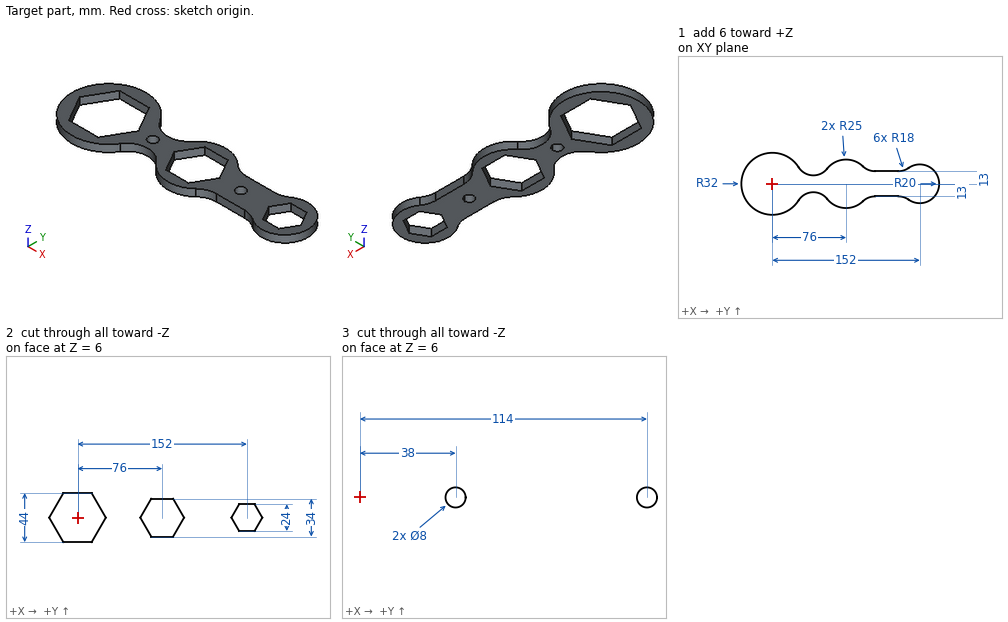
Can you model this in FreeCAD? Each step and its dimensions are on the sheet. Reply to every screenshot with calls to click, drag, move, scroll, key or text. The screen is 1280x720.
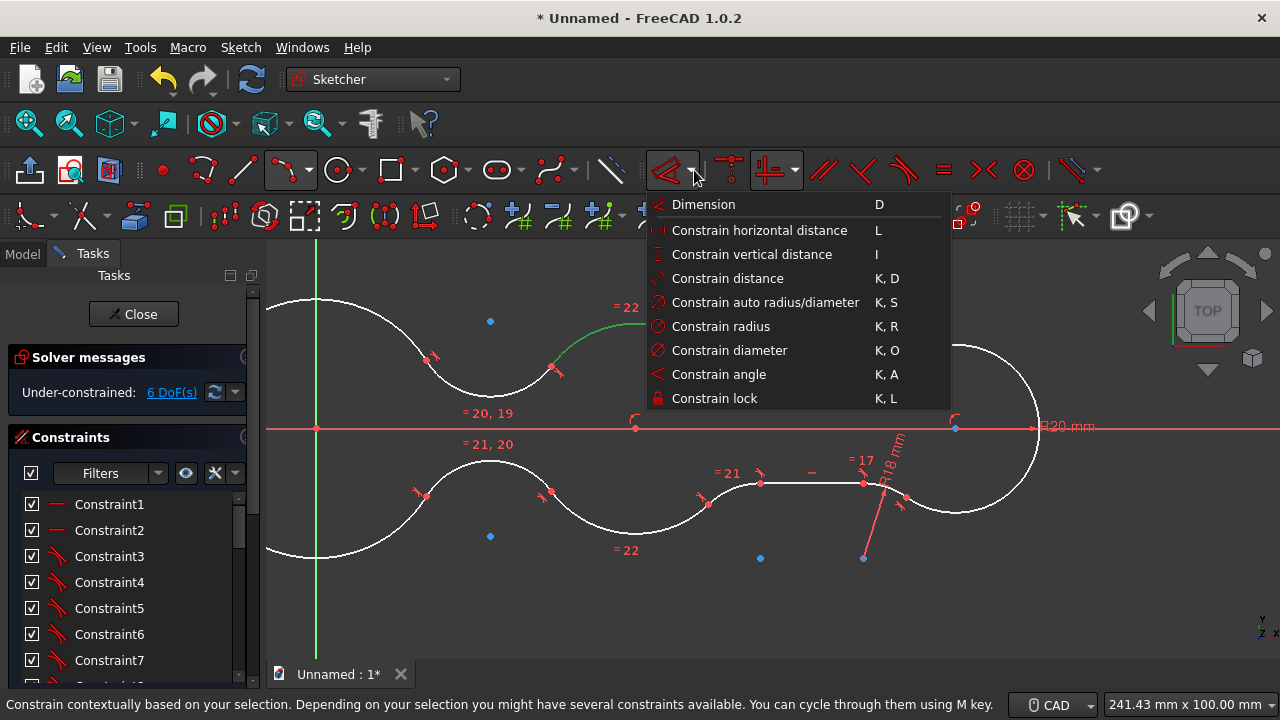
click(799, 326)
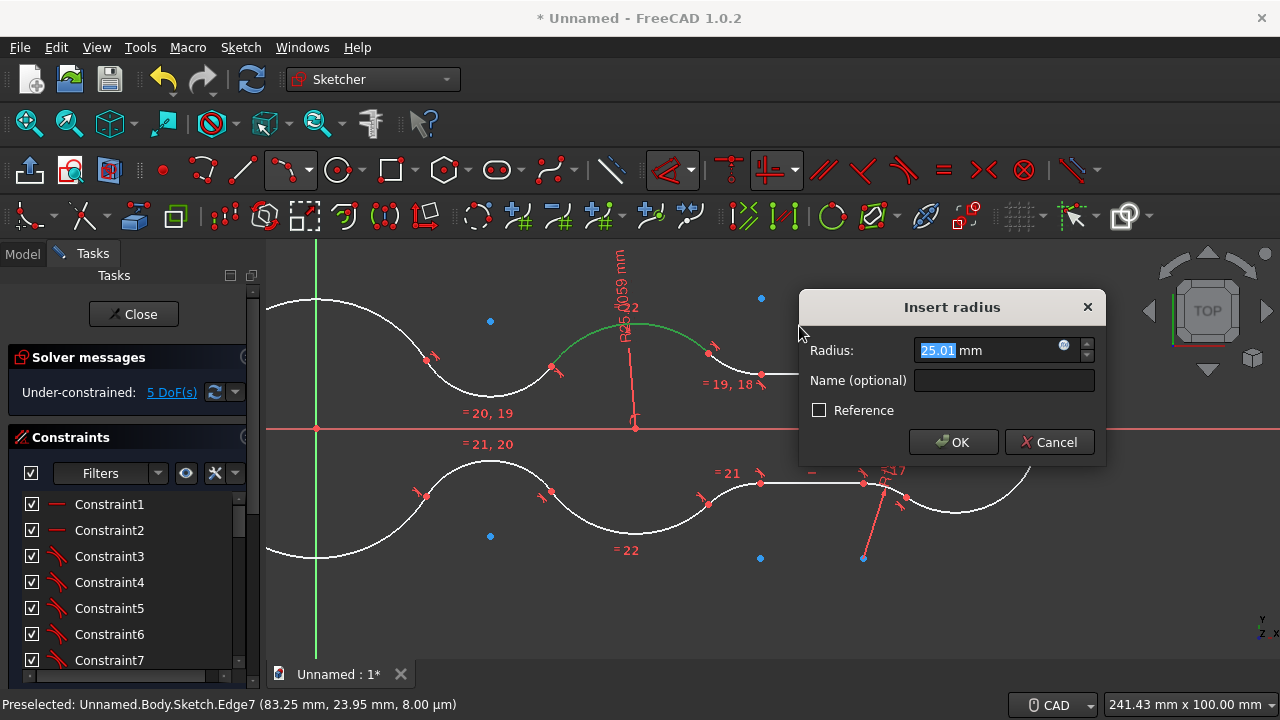
text(25)
key(Return)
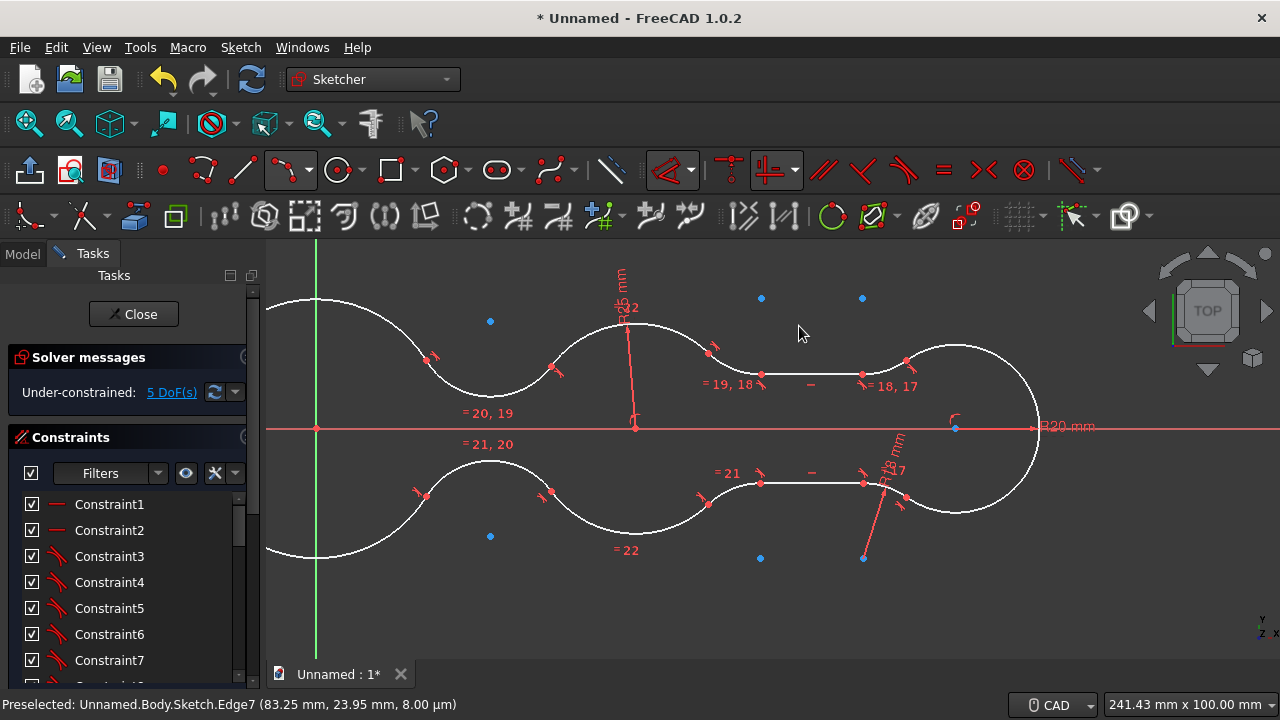
click(314, 299)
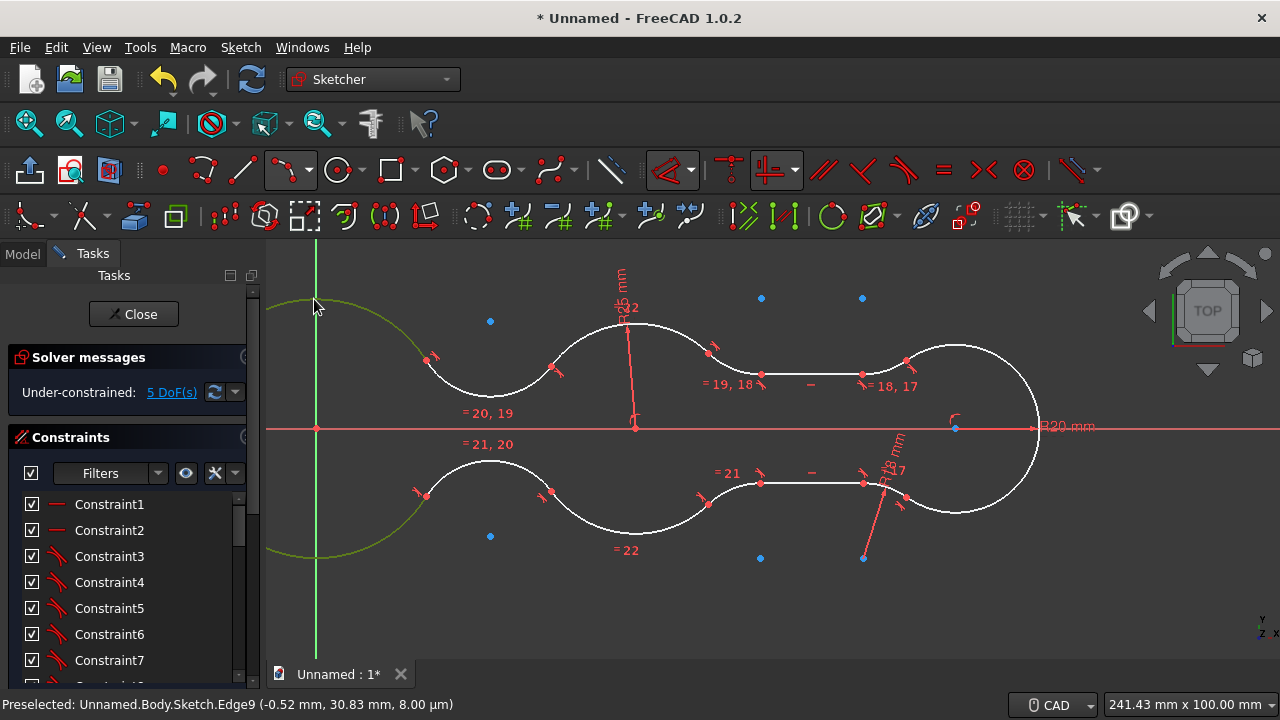
key(k)
key(r)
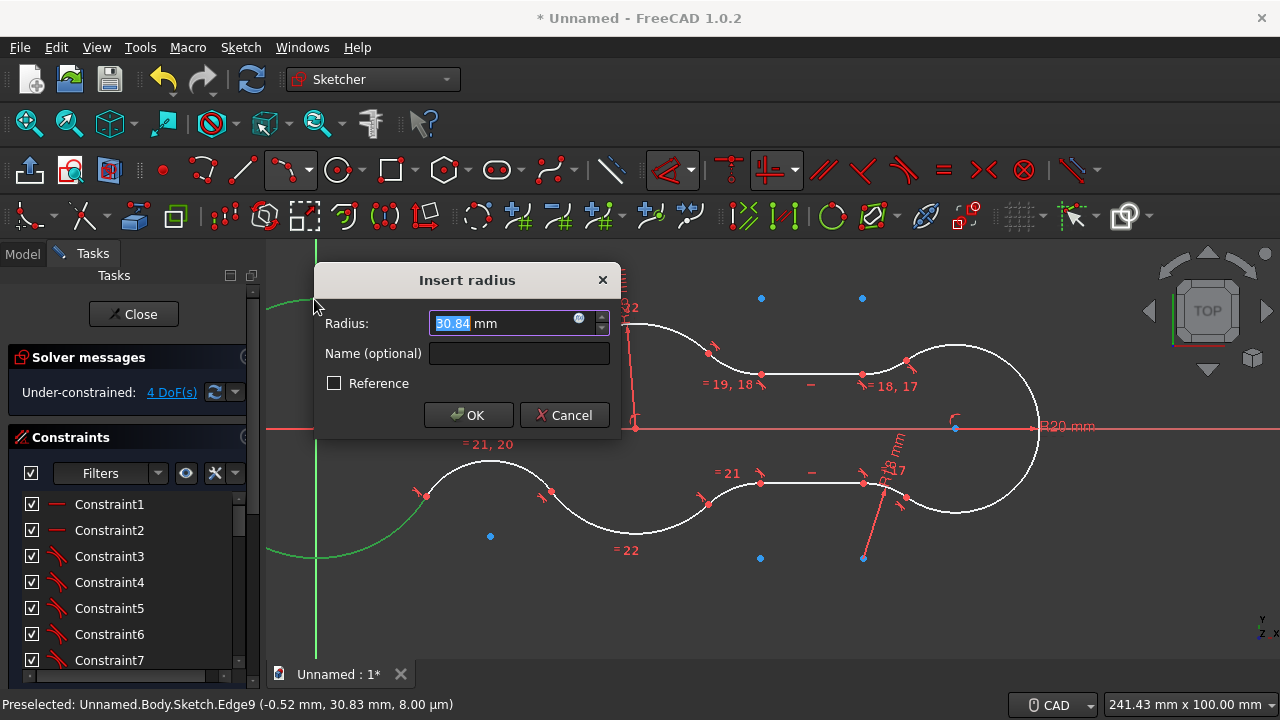
text(32)
key(Return)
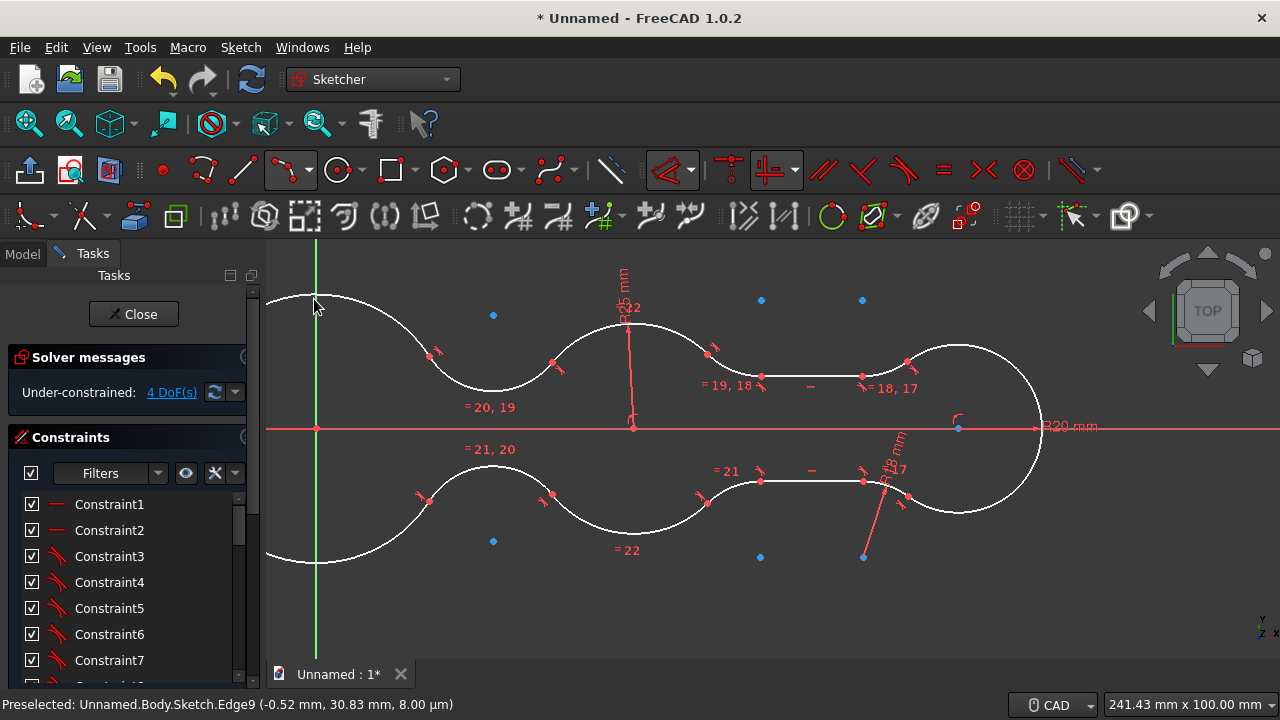
click(761, 481)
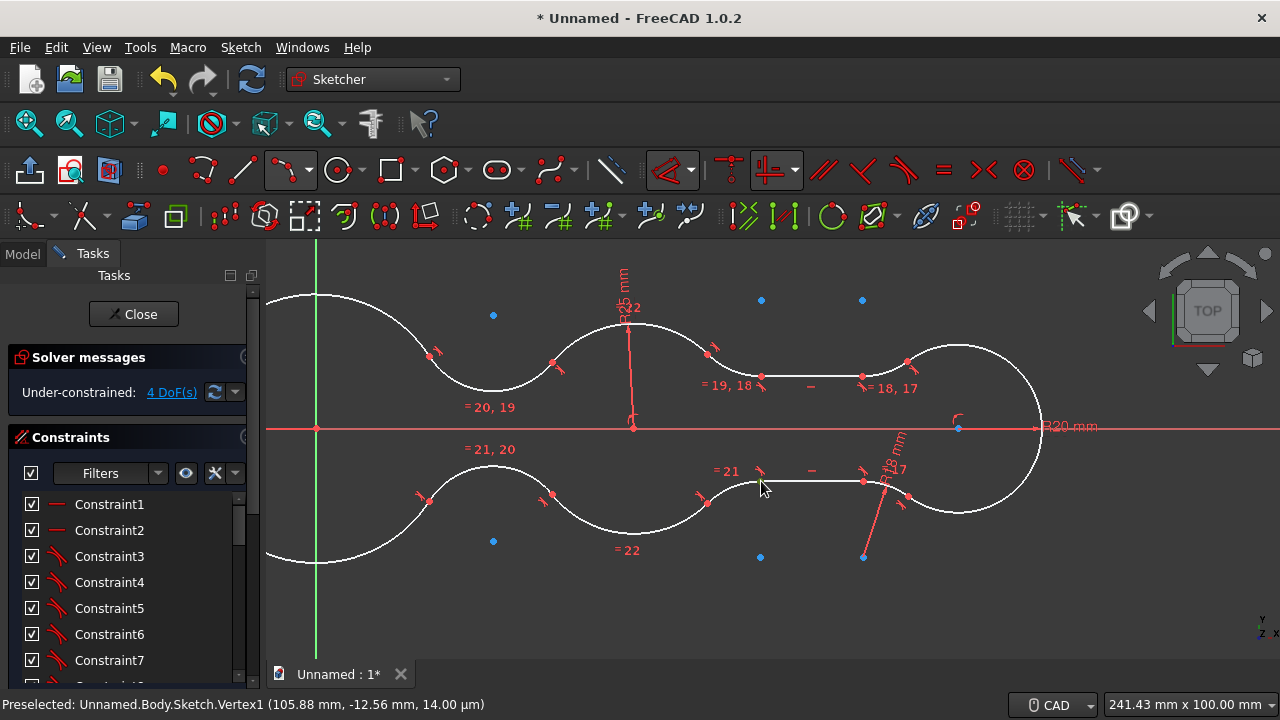
click(694, 170)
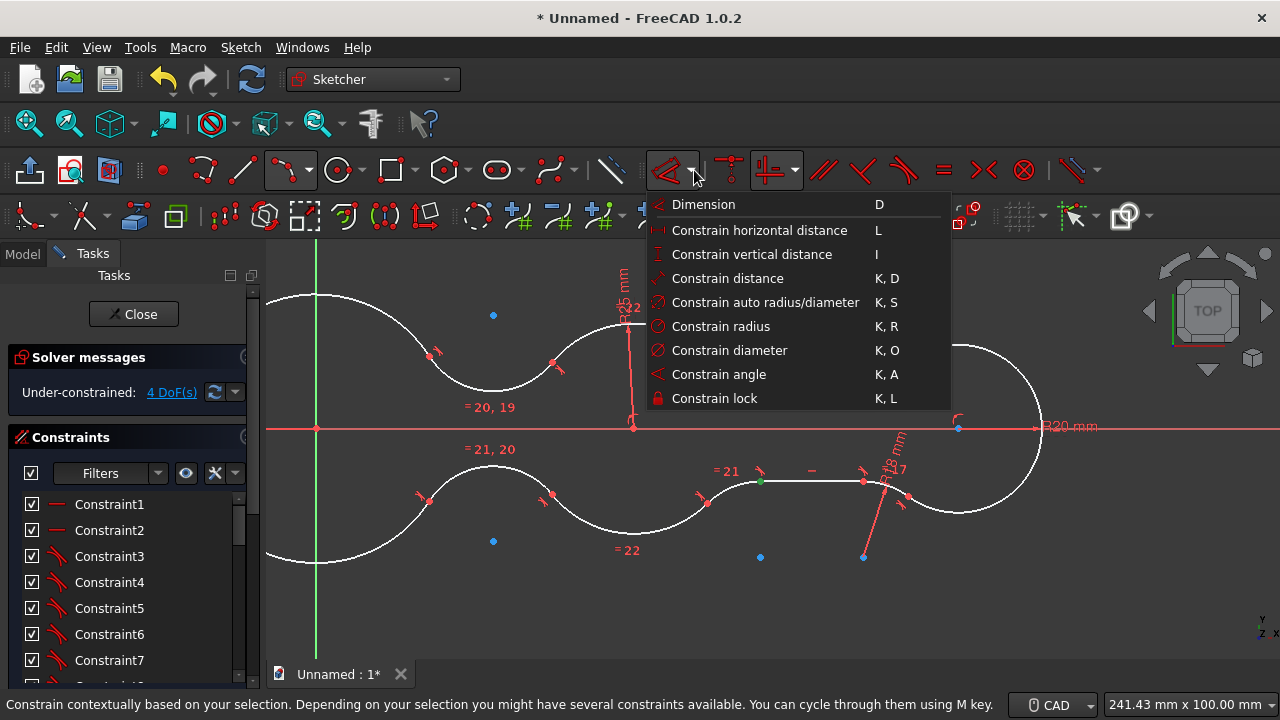
click(799, 254)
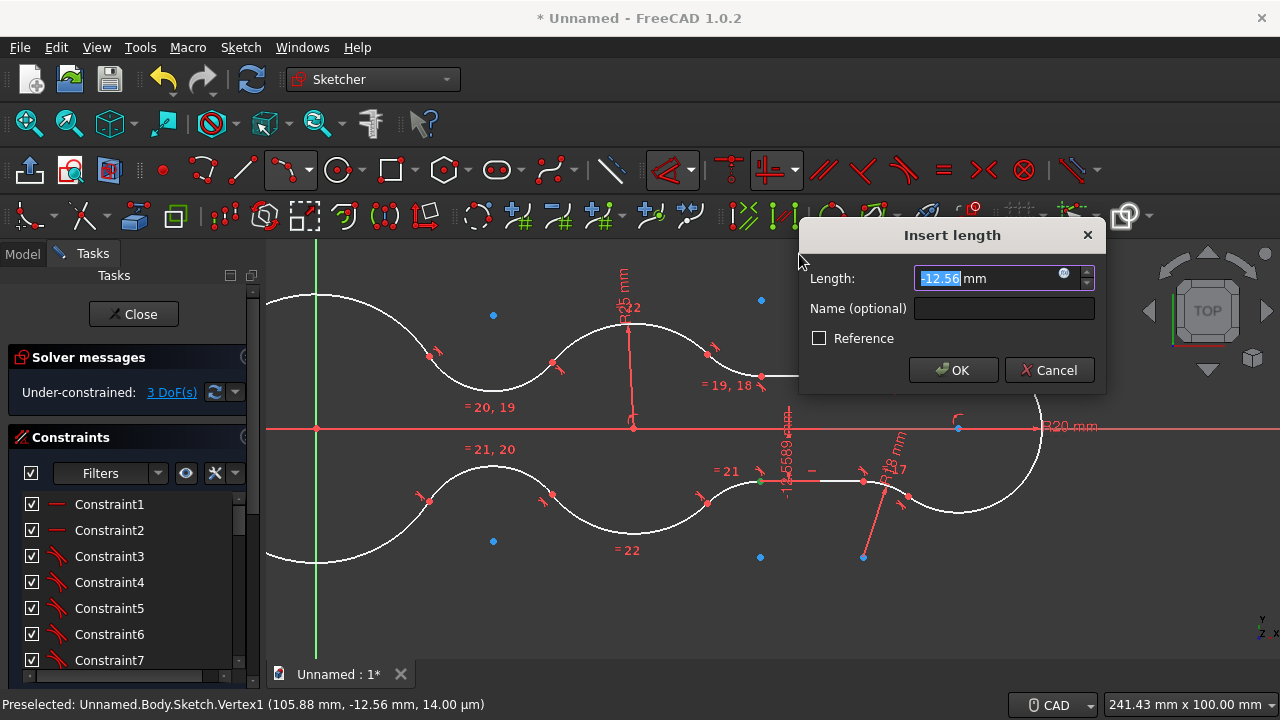
text(-13)
key(Return)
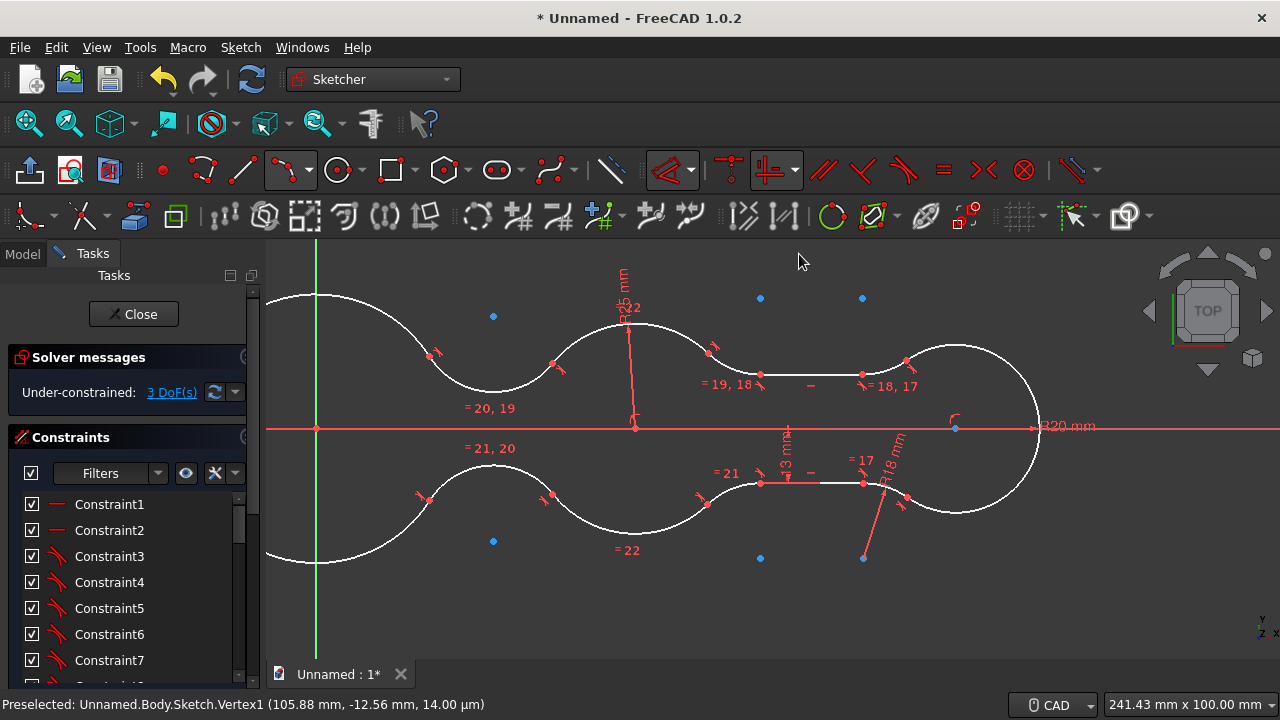
click(863, 375)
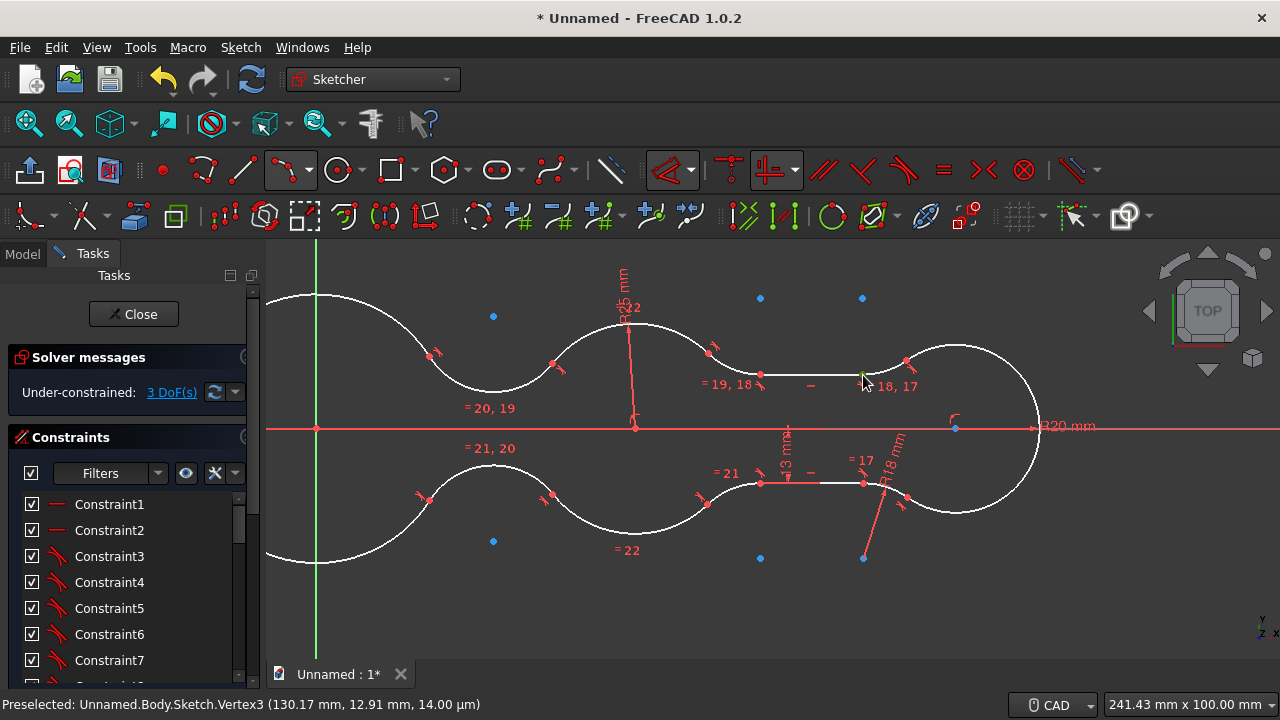
click(694, 170)